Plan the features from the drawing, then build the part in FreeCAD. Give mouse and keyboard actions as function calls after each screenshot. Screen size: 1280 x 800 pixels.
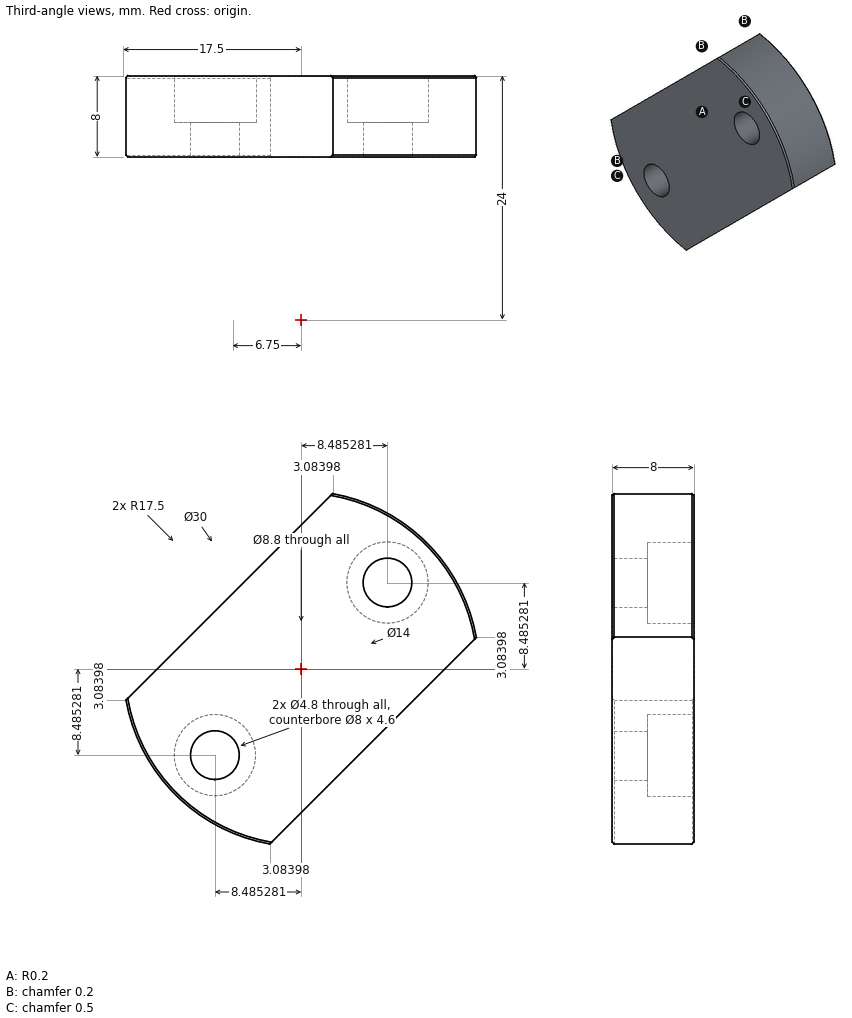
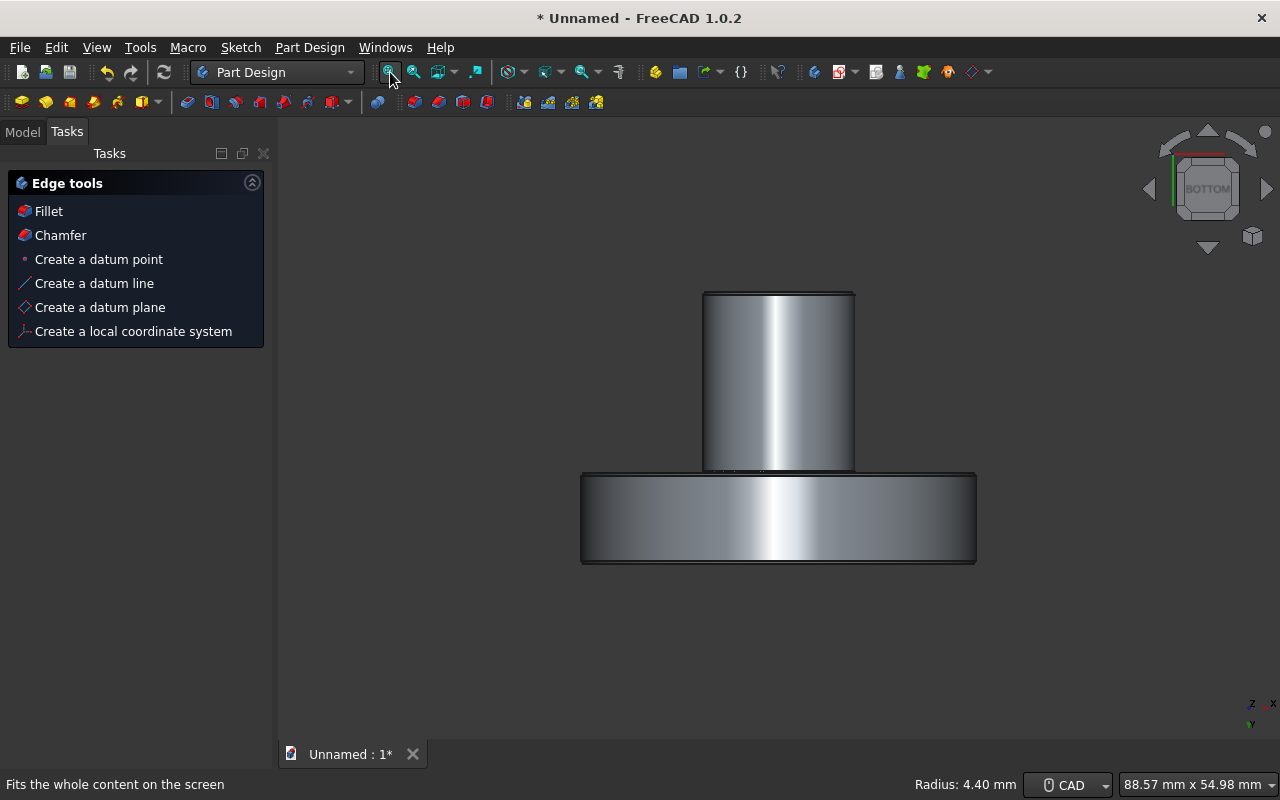
key(4)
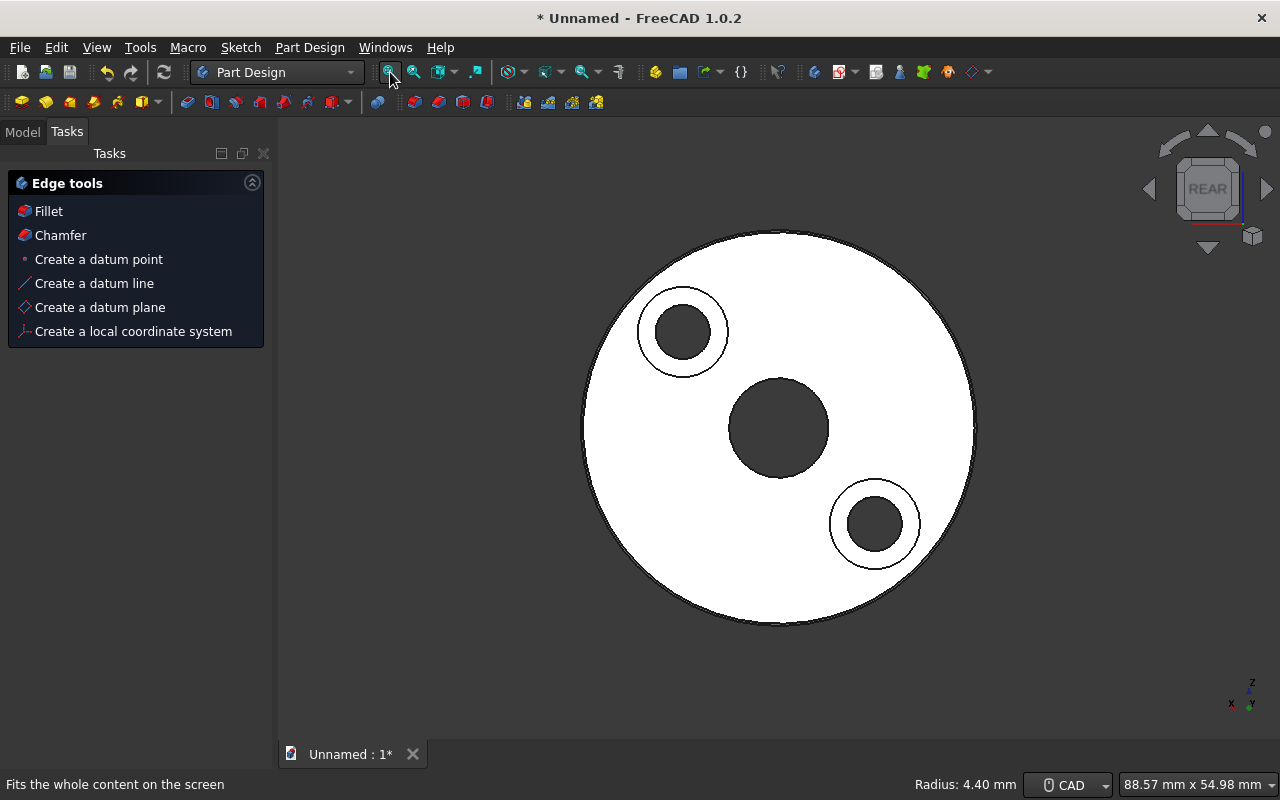
click(829, 427, ctrl)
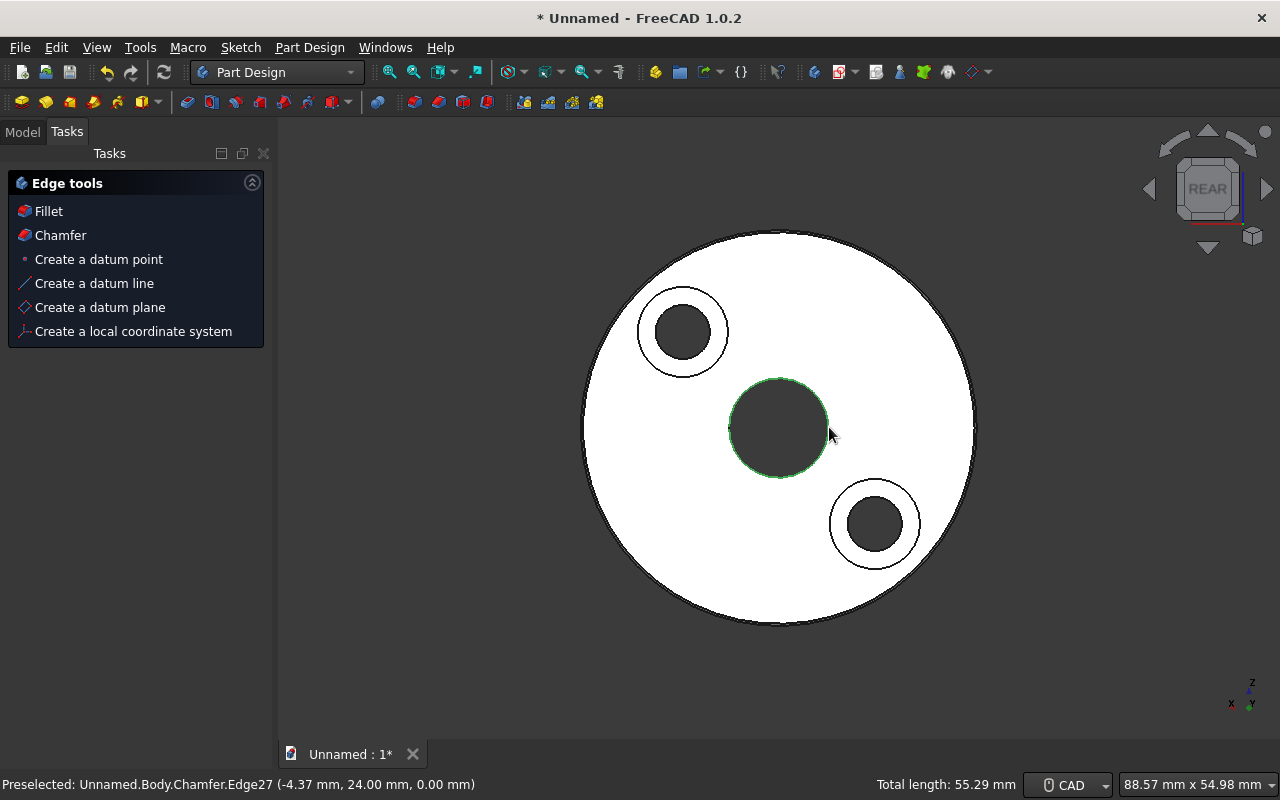
click(440, 102)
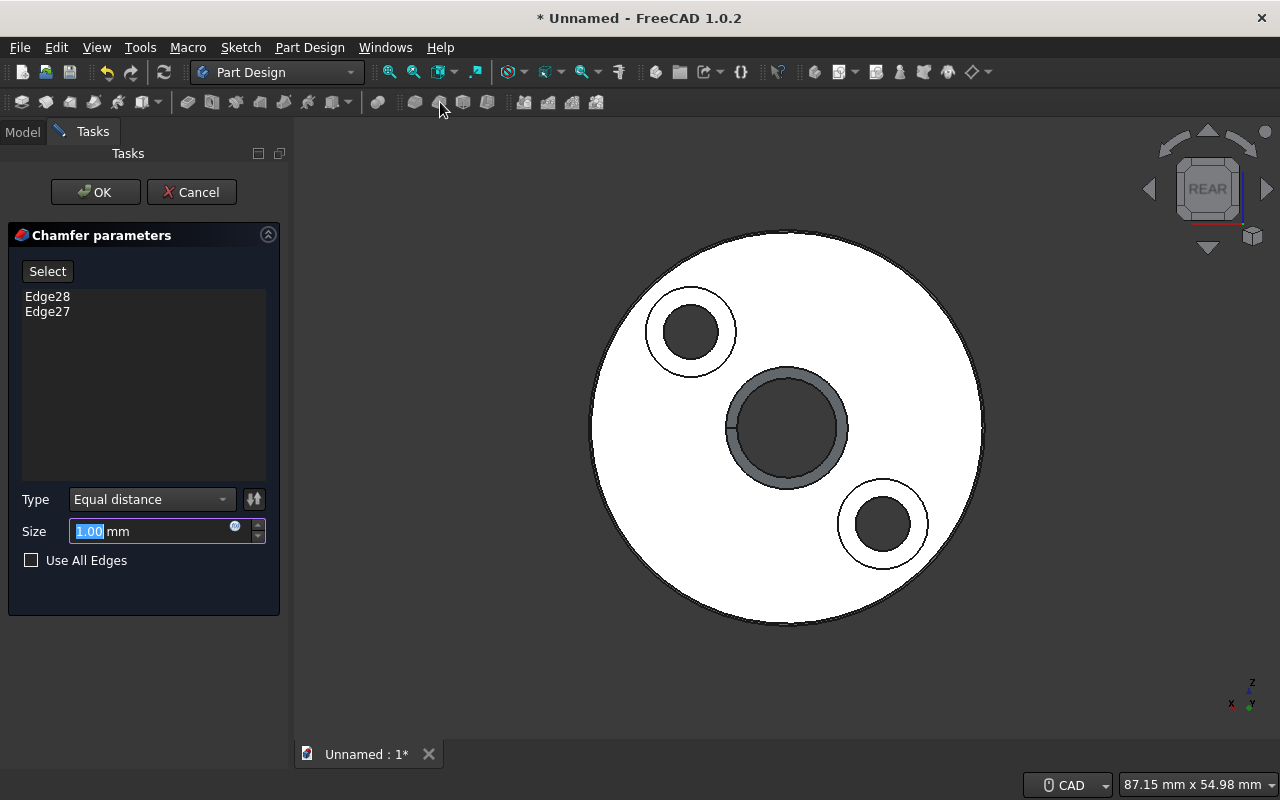
text(0.5)
key(Tab)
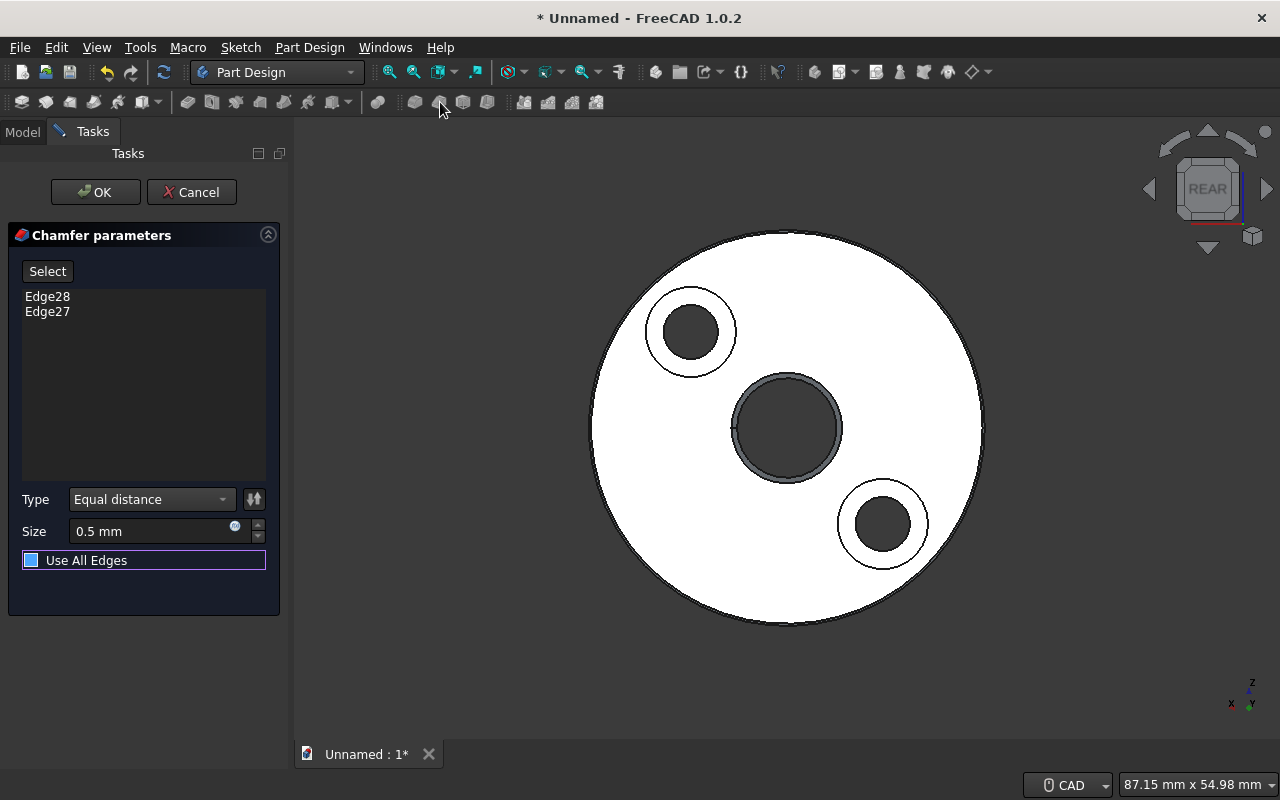
click(96, 192)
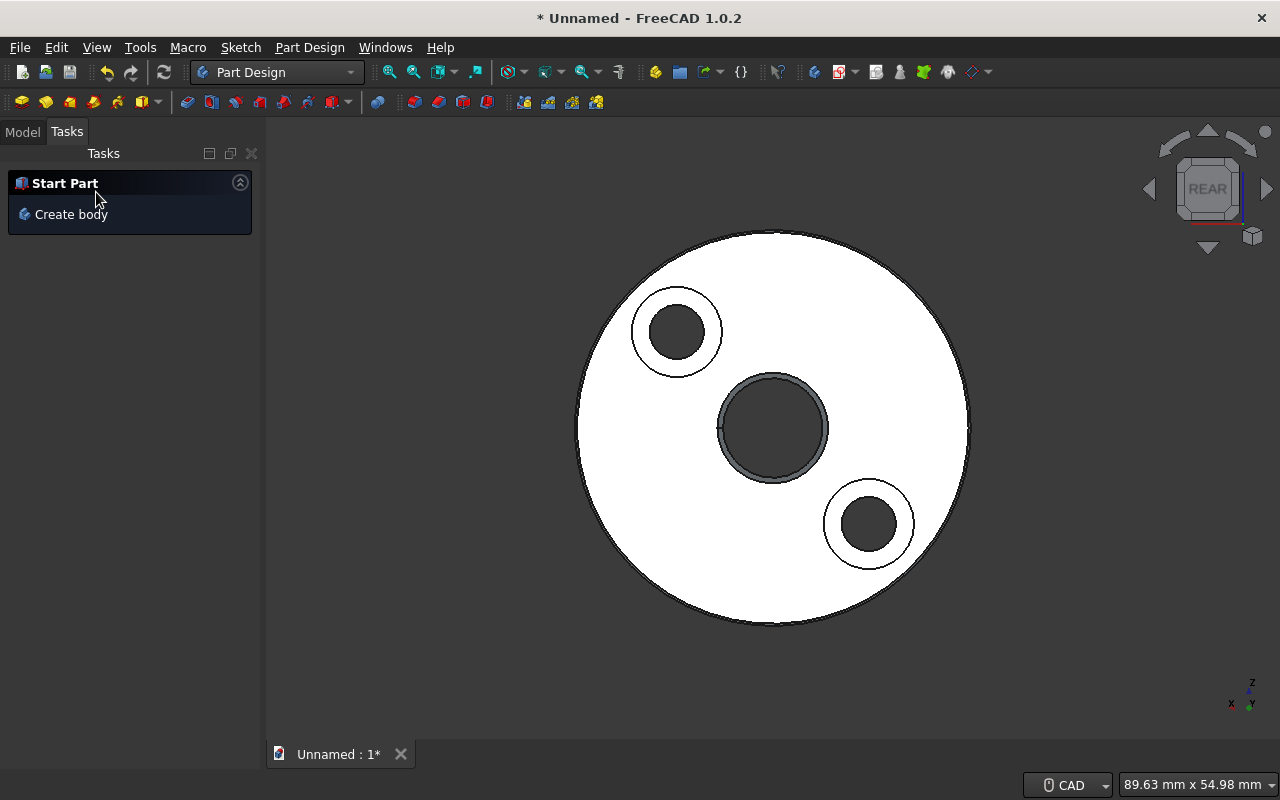
click(661, 483)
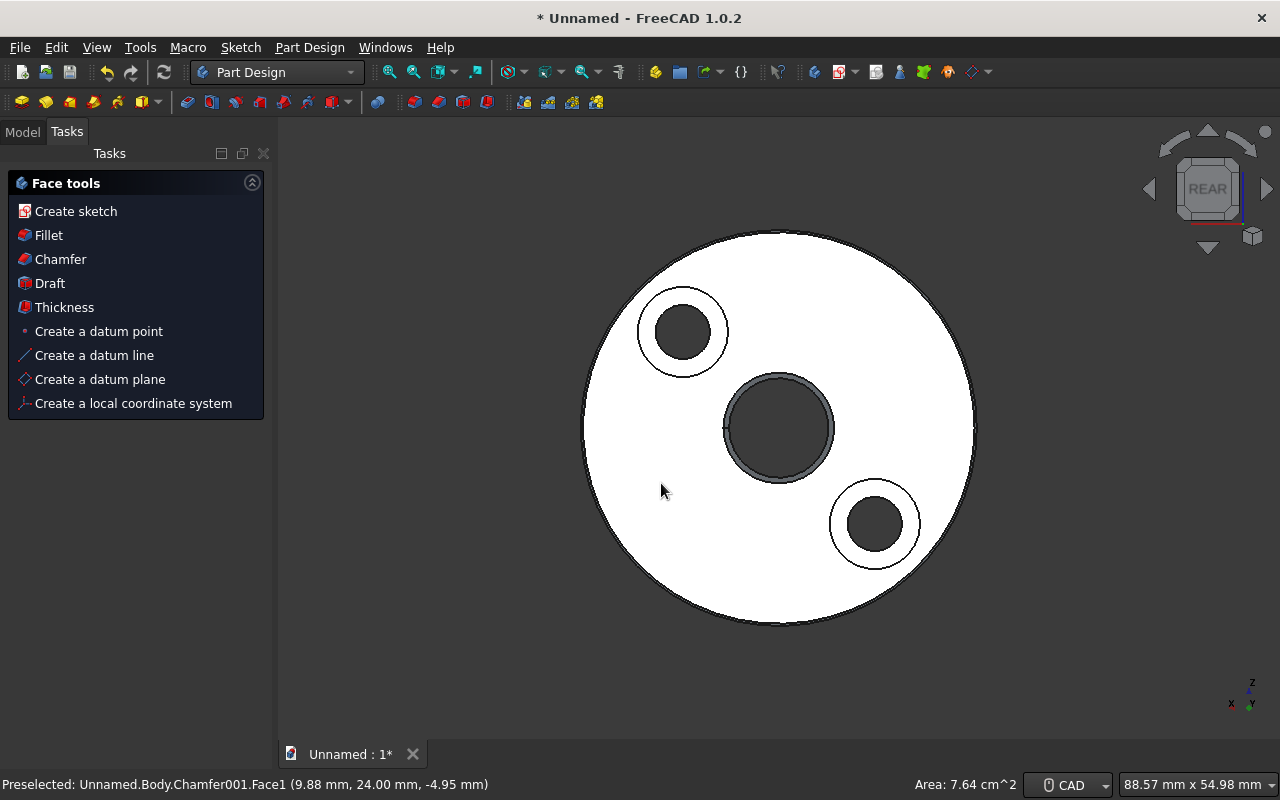
click(840, 72)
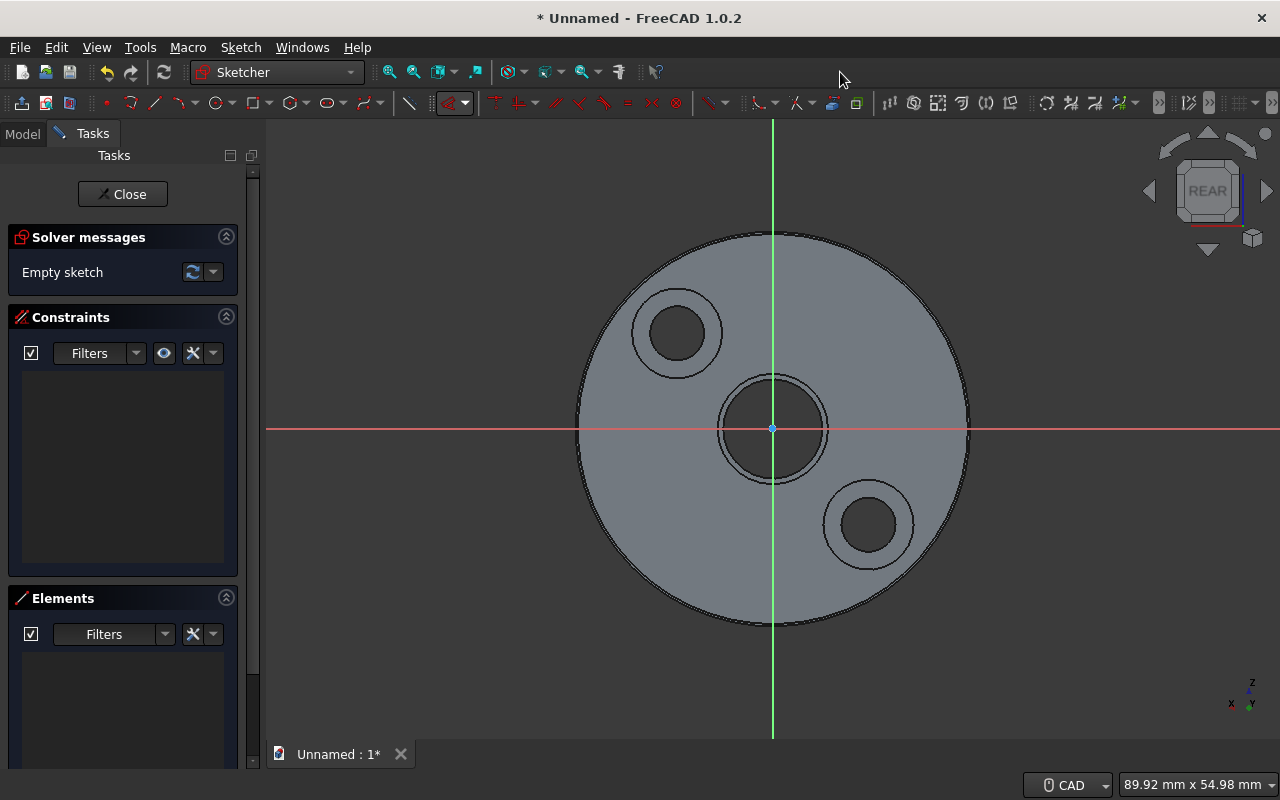
click(156, 104)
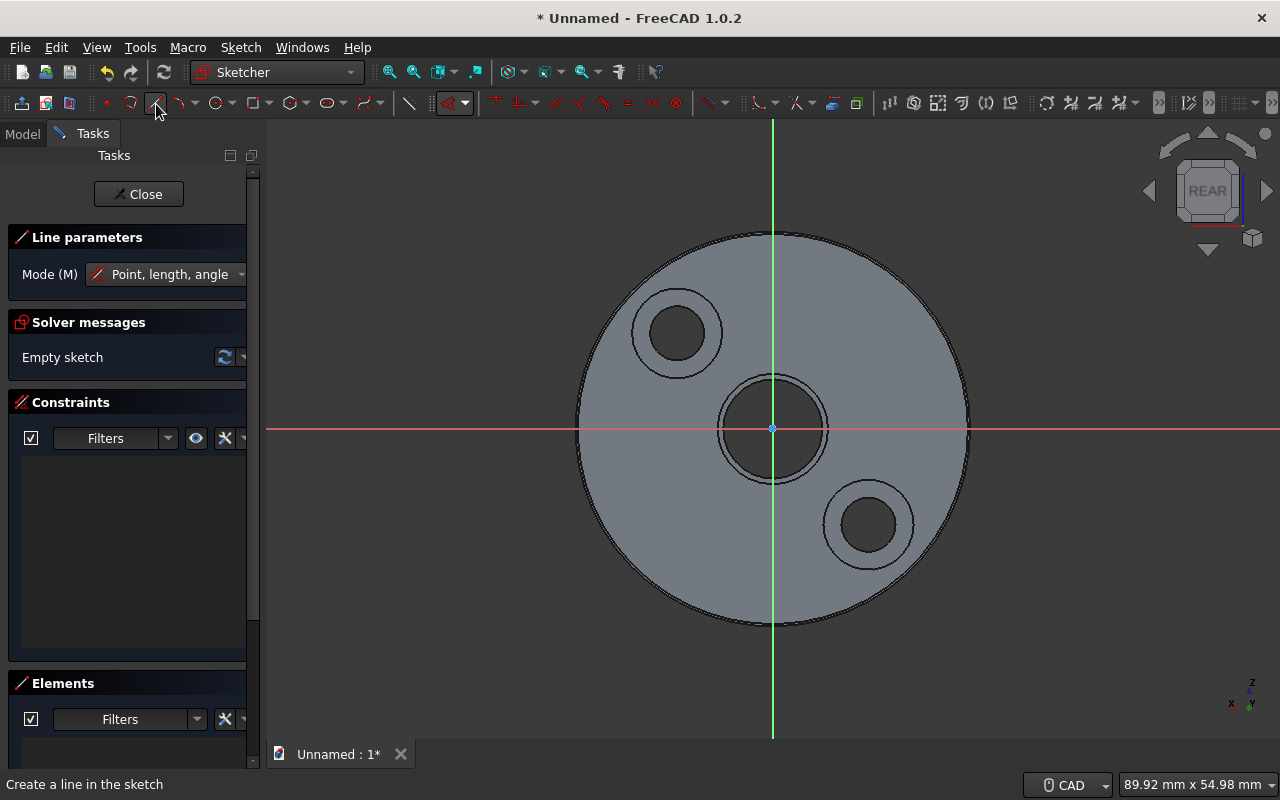
click(738, 235)
click(967, 464)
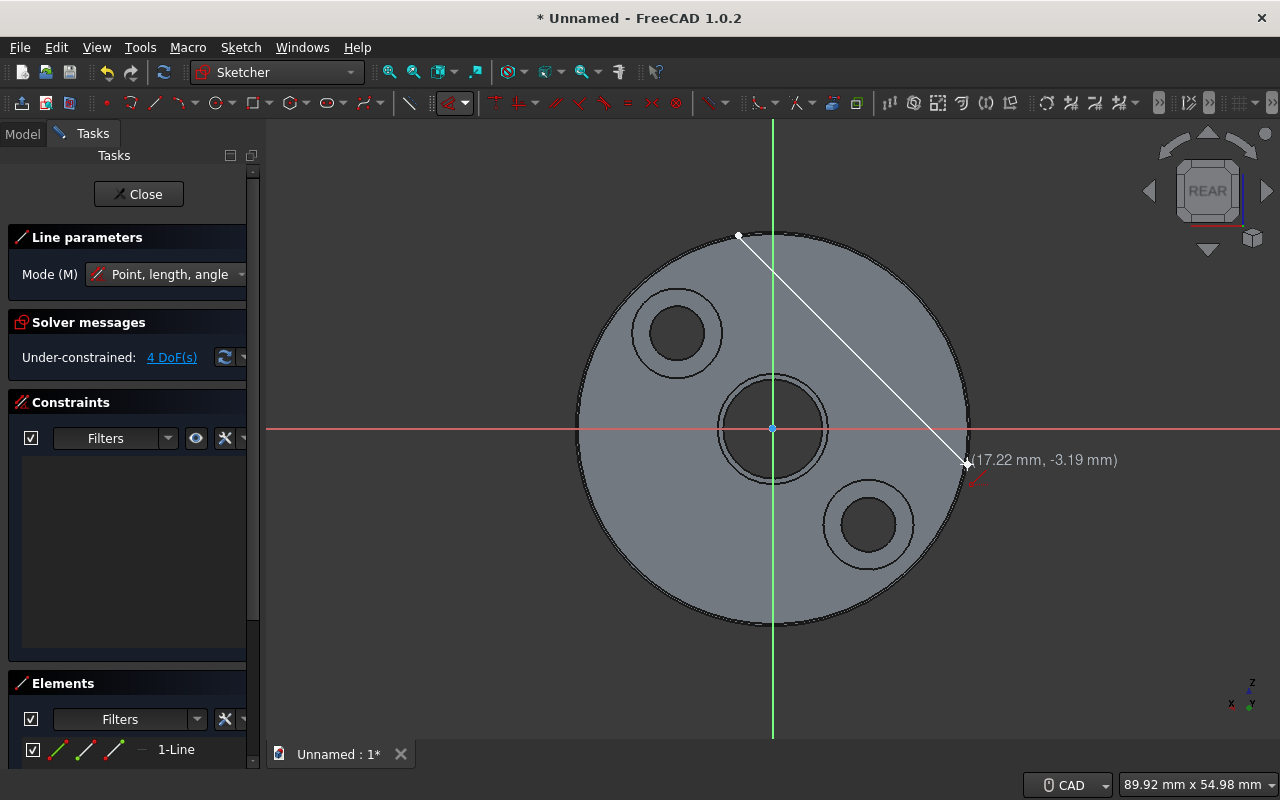
click(180, 104)